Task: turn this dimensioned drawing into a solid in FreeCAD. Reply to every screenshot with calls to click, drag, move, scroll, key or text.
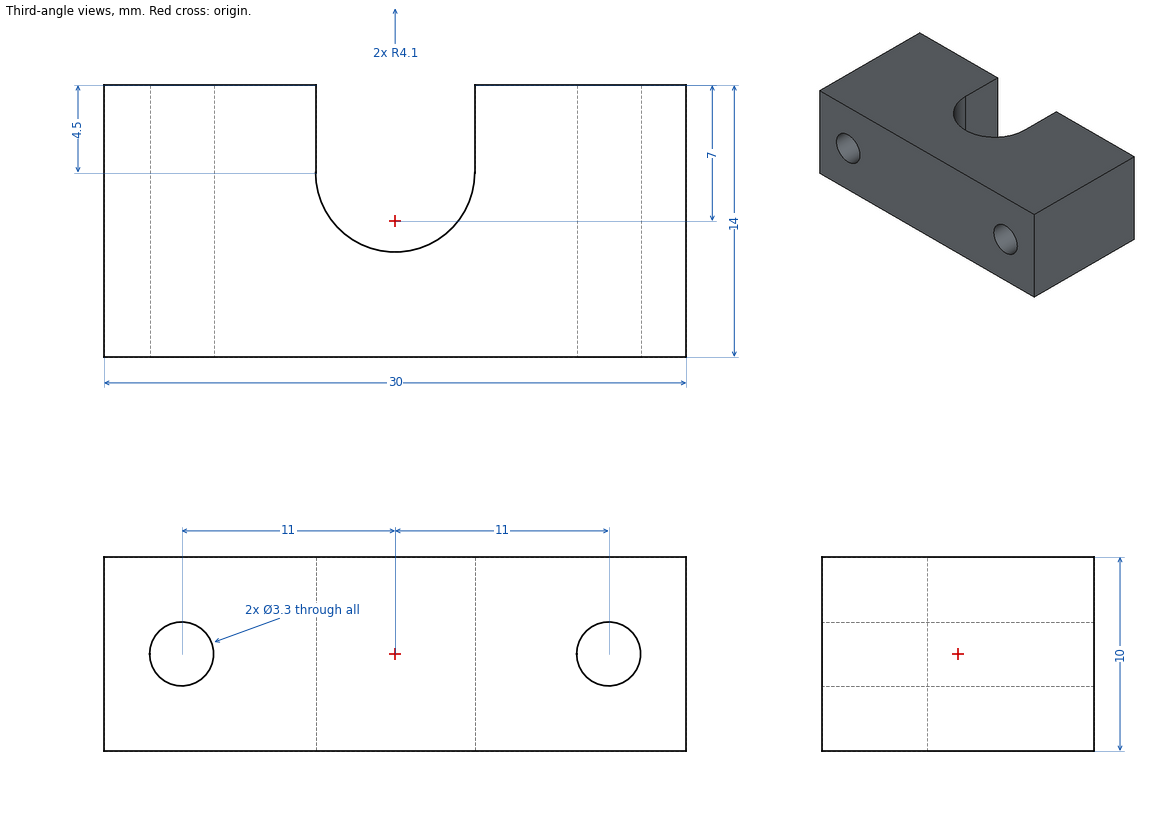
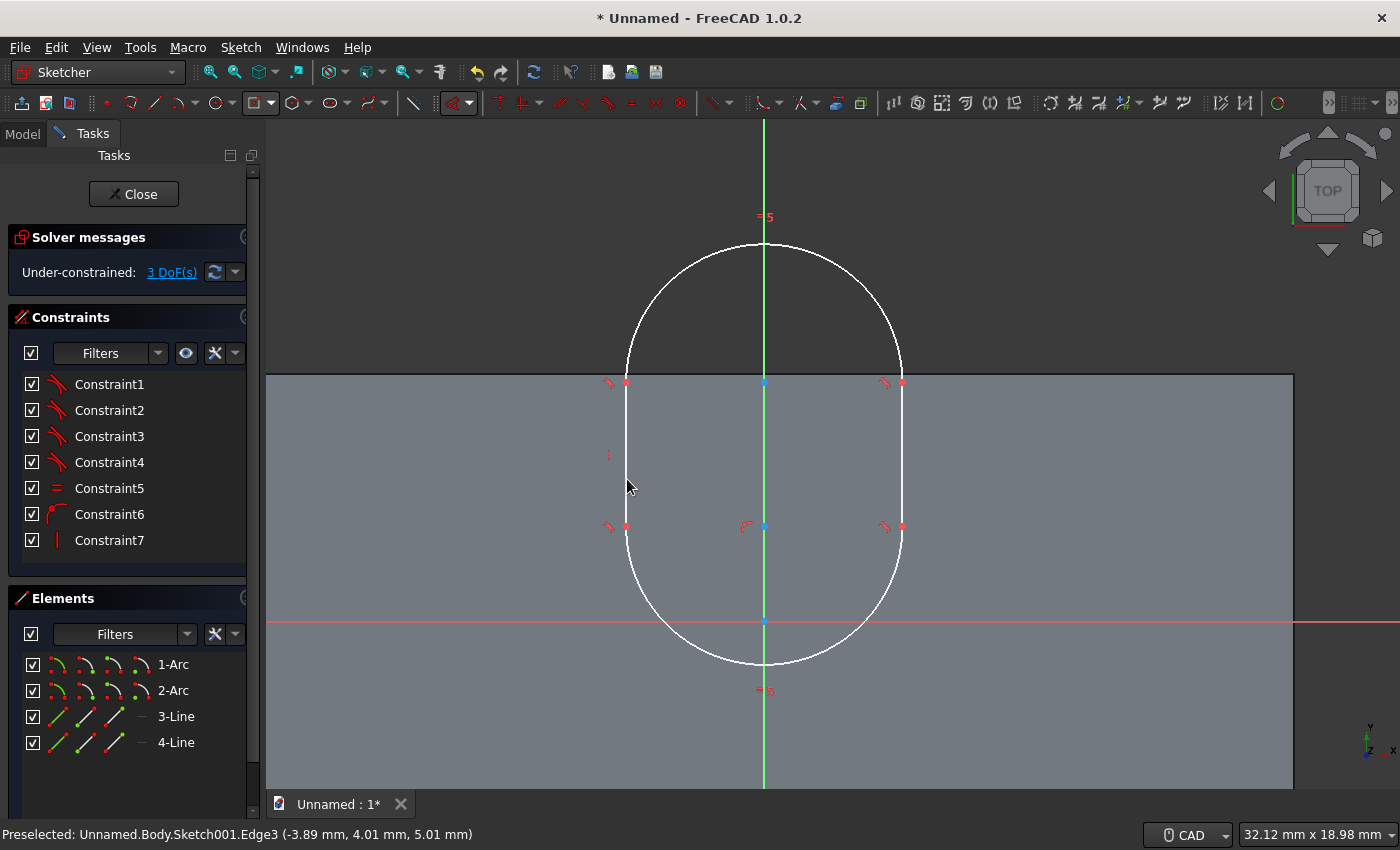
click(683, 639)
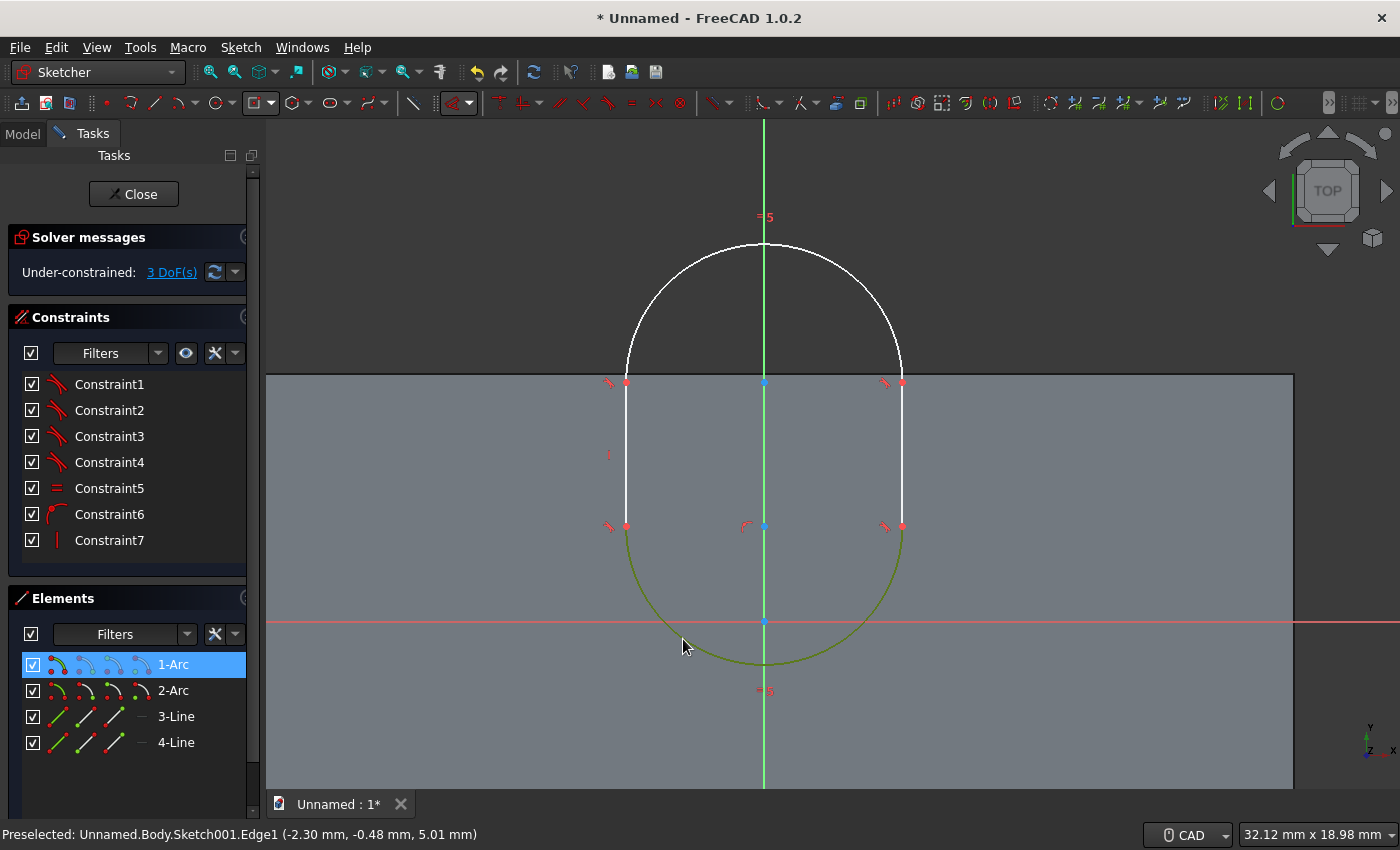
click(472, 104)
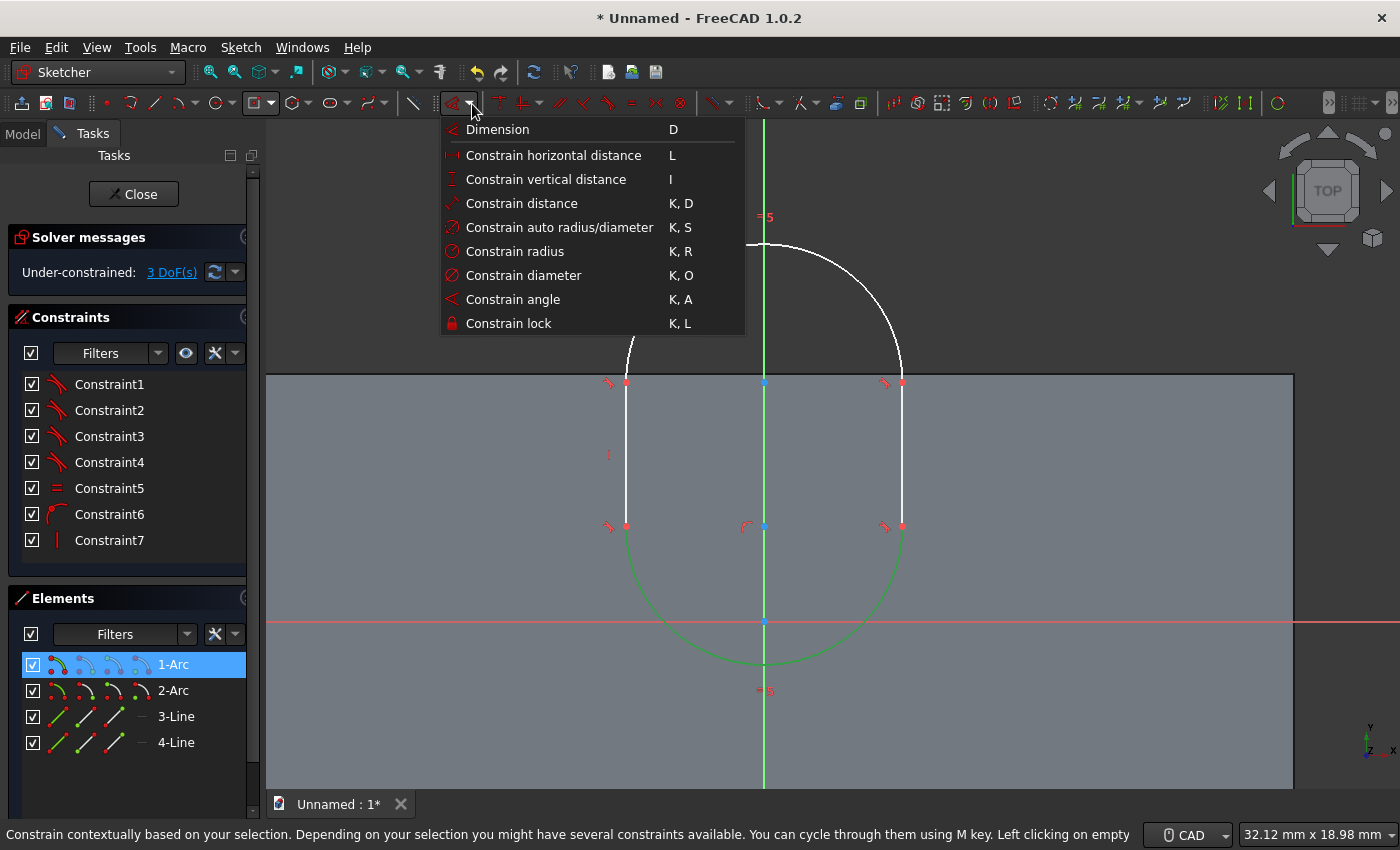
click(593, 251)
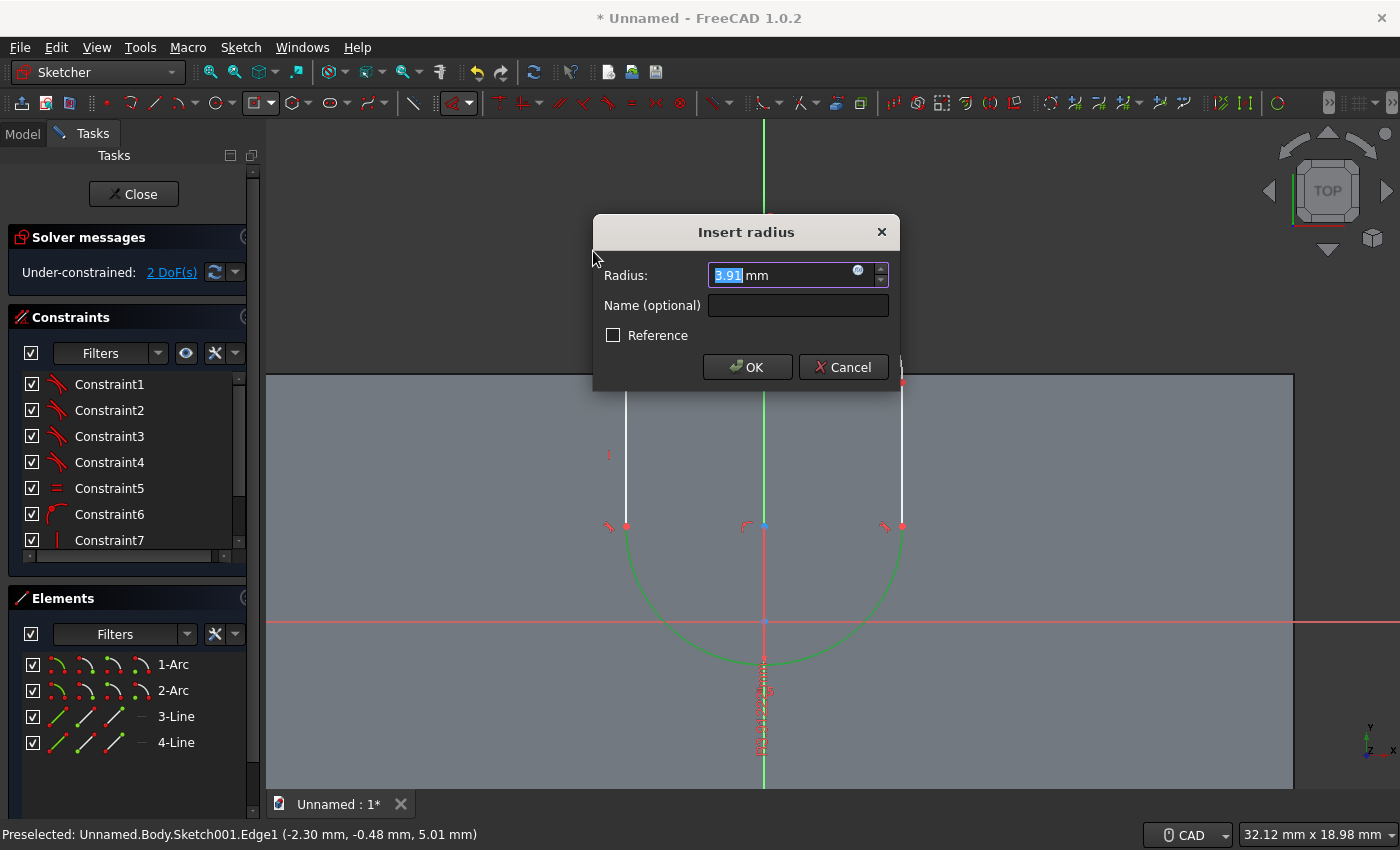
text(4.1)
key(Return)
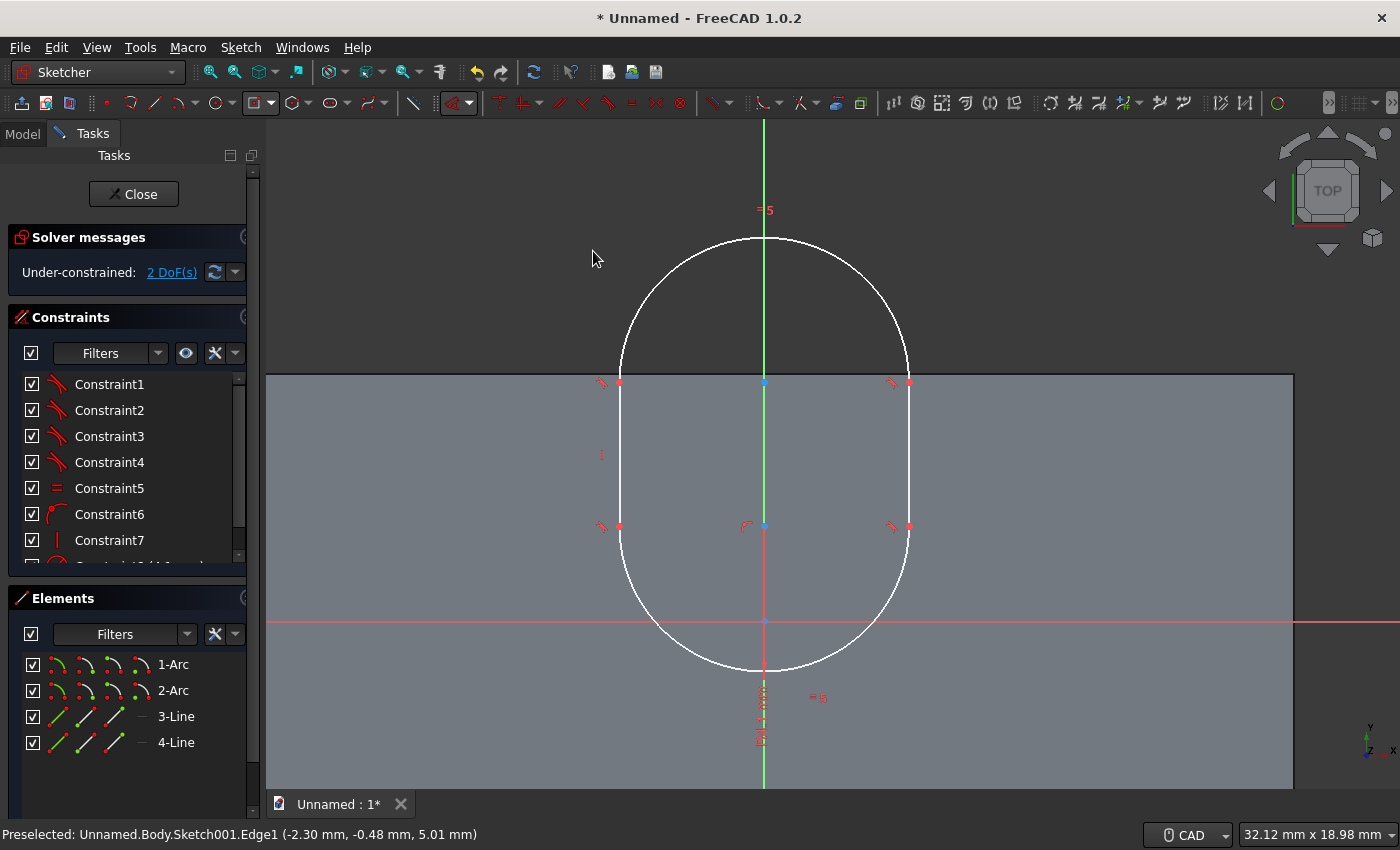
click(909, 382)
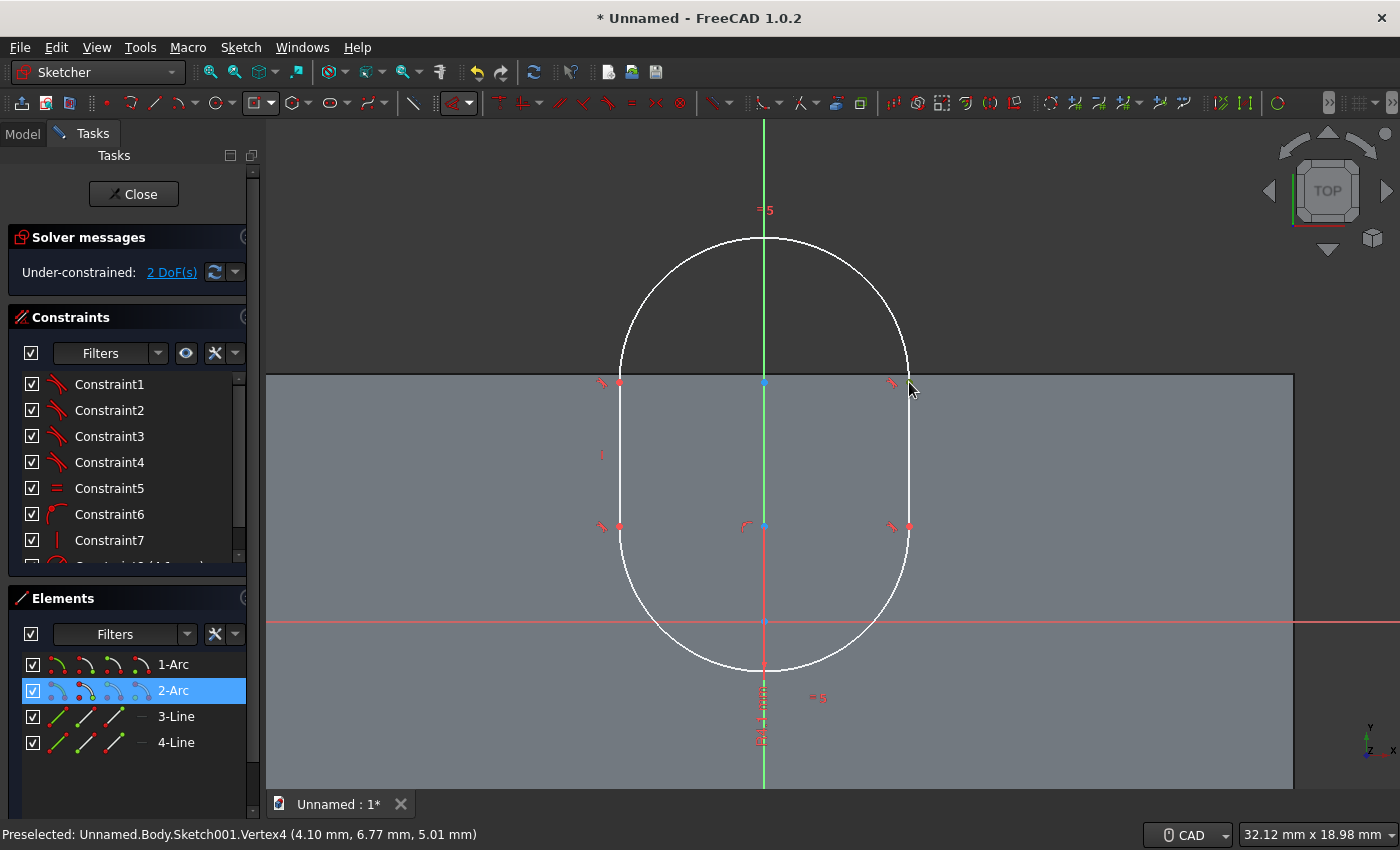
key(i)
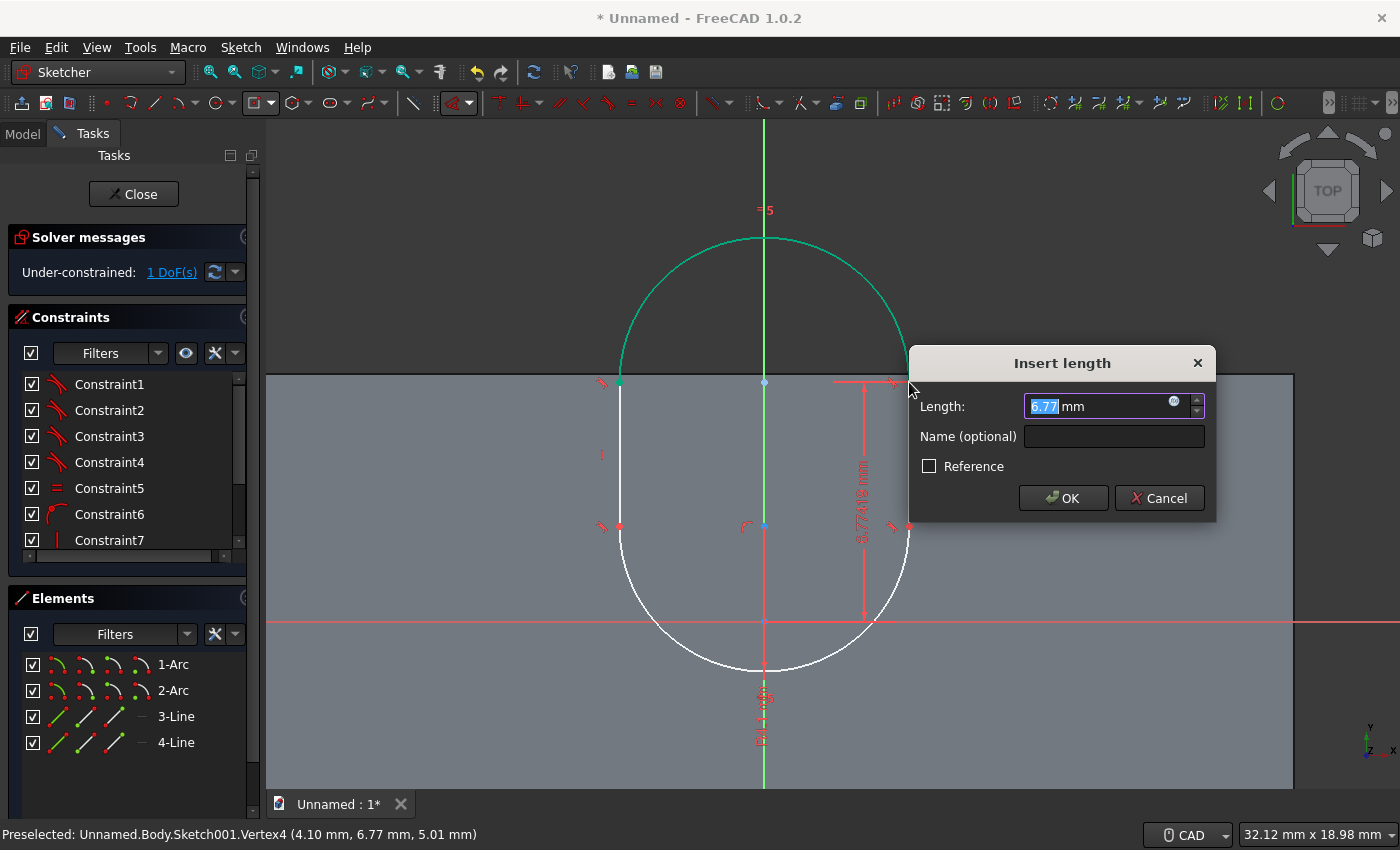
text(7)
key(Return)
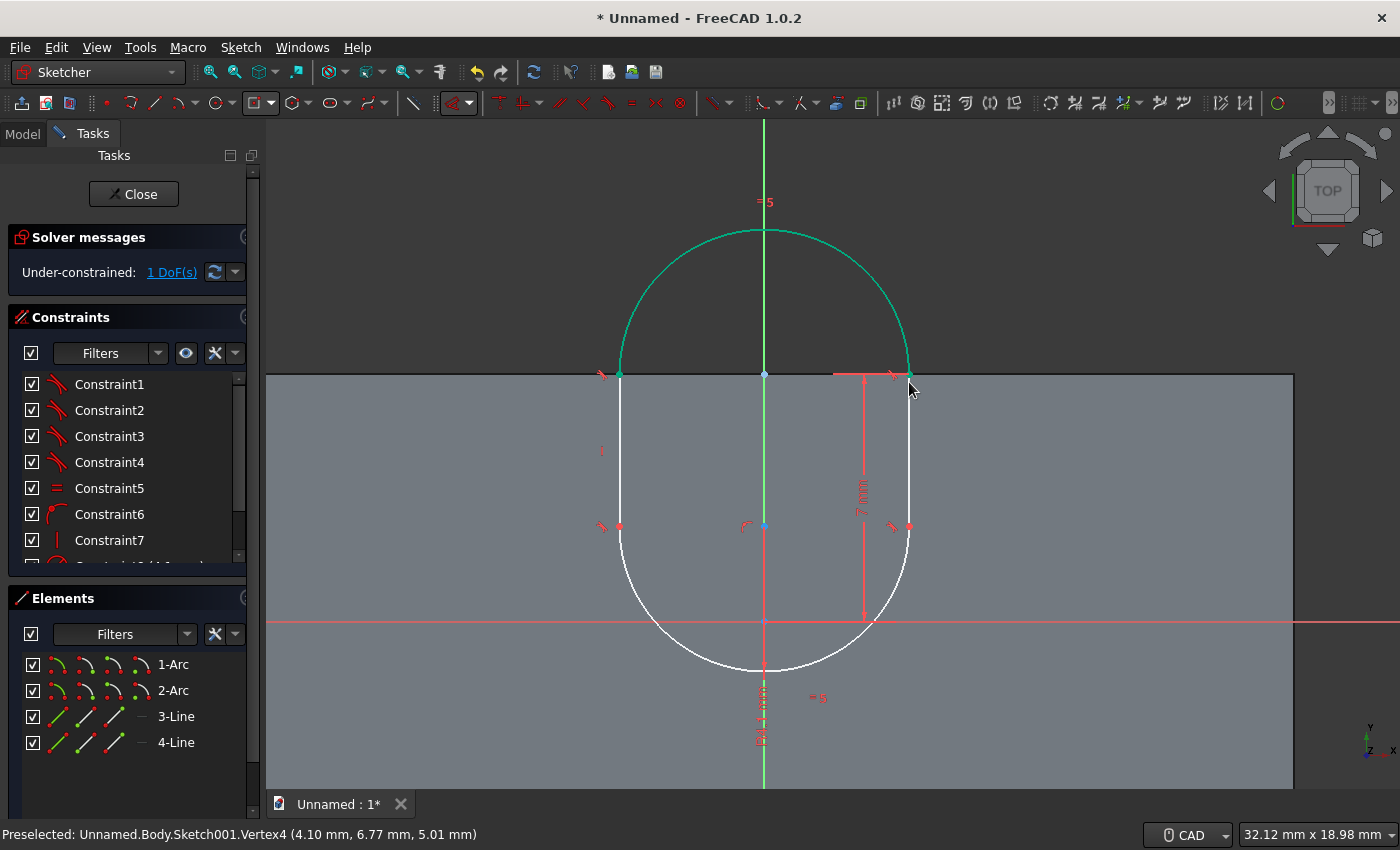
click(620, 481)